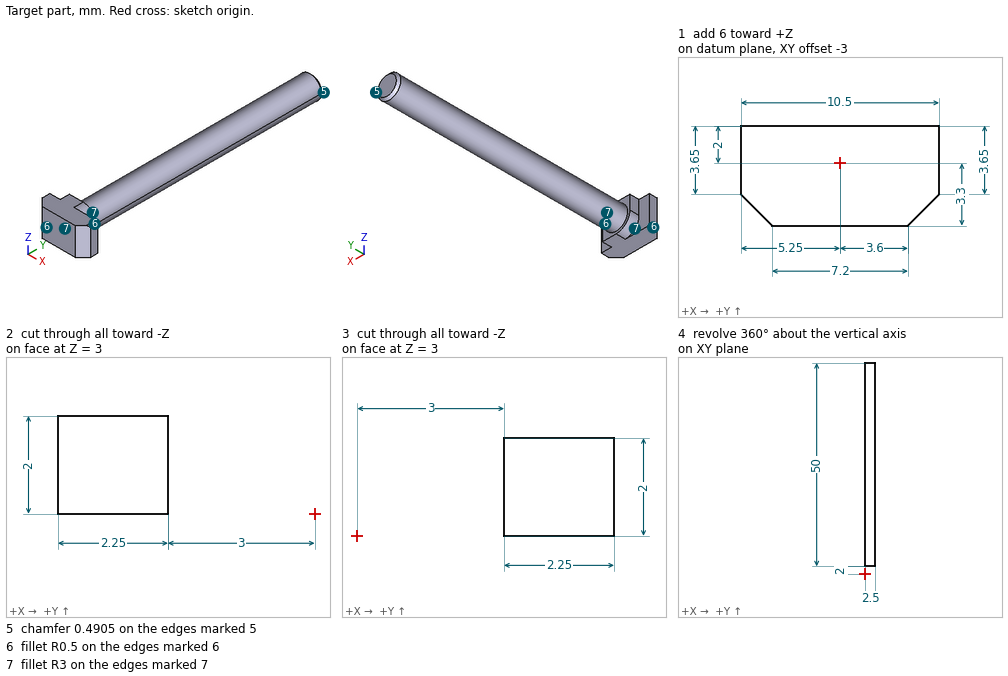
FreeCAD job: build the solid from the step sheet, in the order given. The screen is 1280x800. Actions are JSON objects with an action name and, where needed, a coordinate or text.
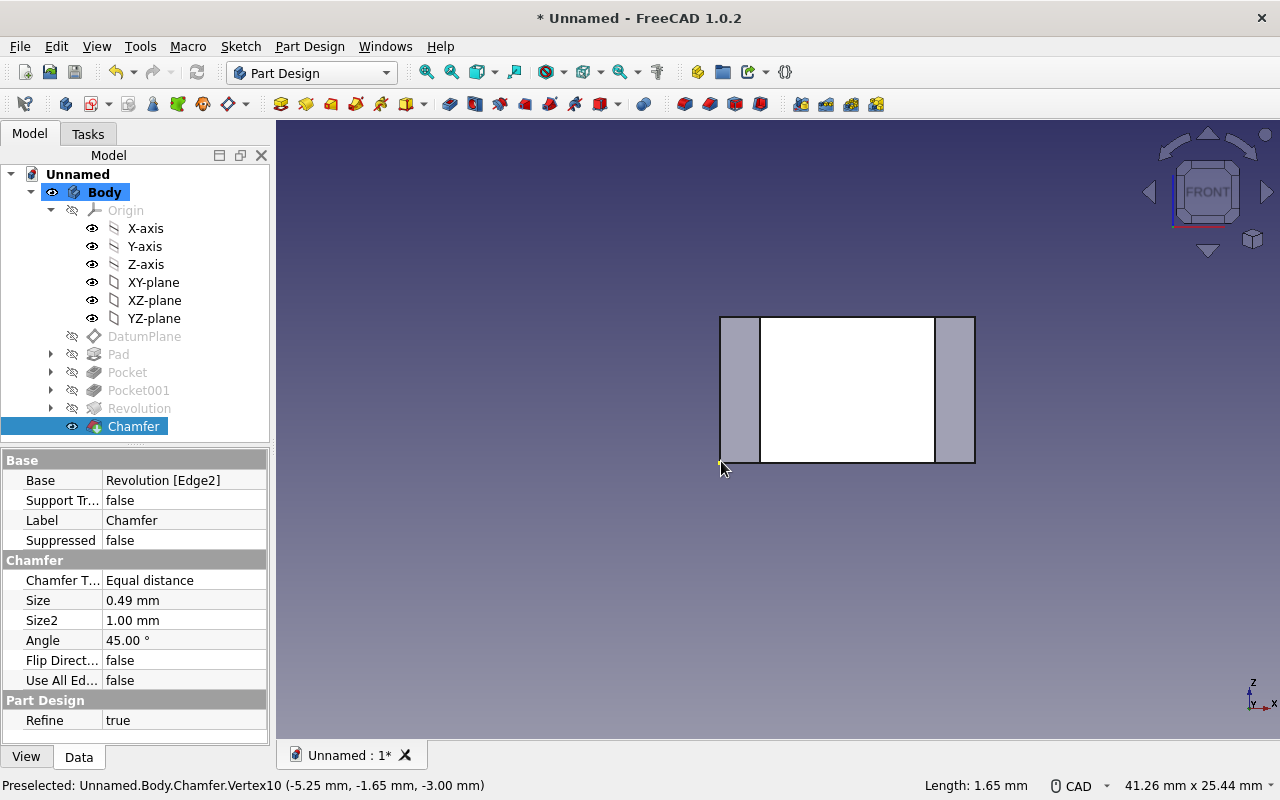
{"action": "key", "text": "v f"}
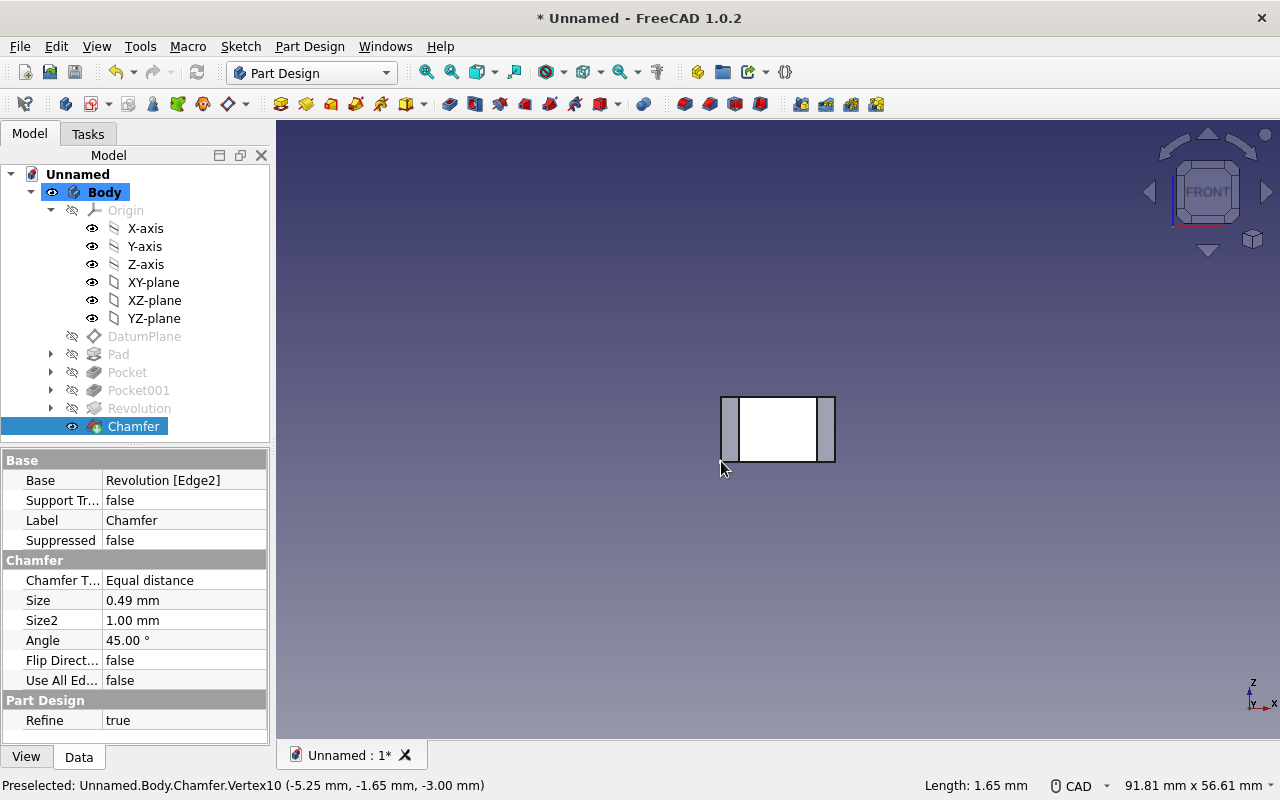
{"action": "key", "text": "3"}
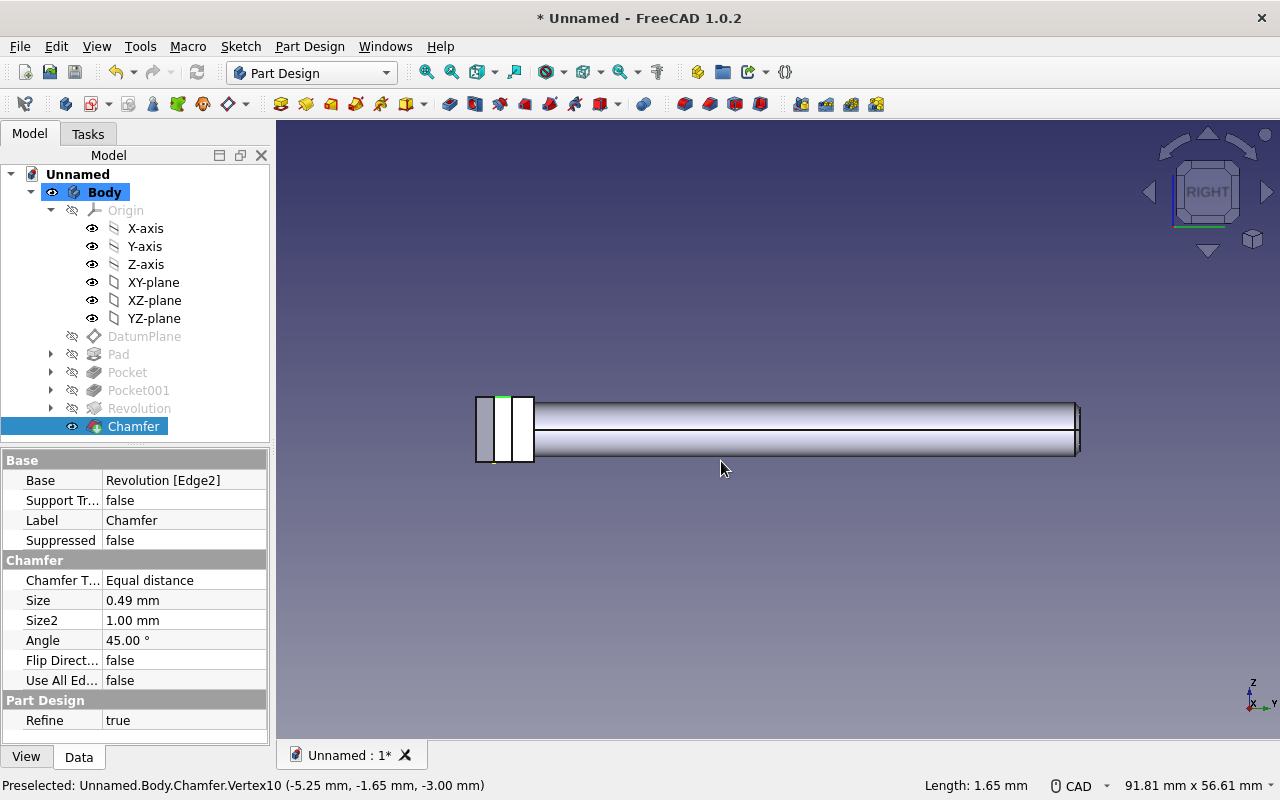
{"action": "scroll", "coordinate": [503, 461], "scroll_direction": "up", "scroll_amount": 4}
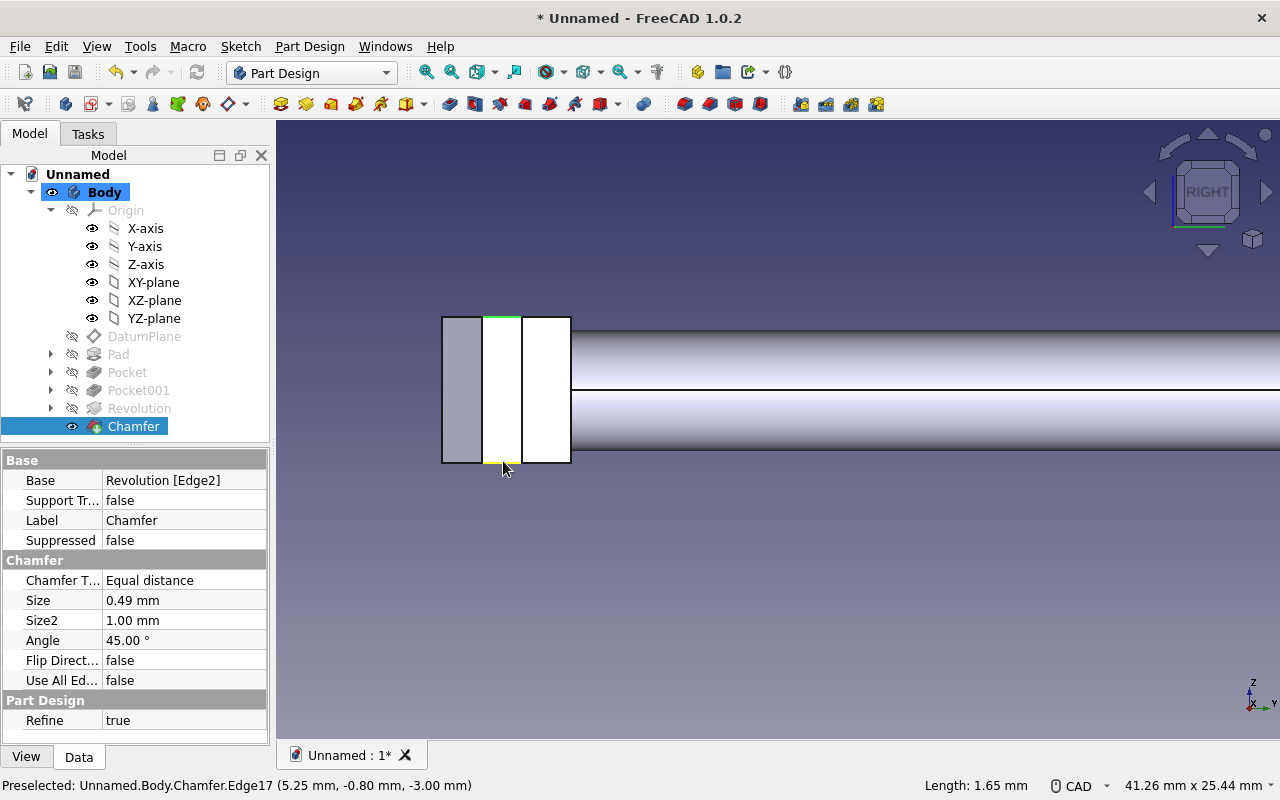
{"action": "key", "text": "v f"}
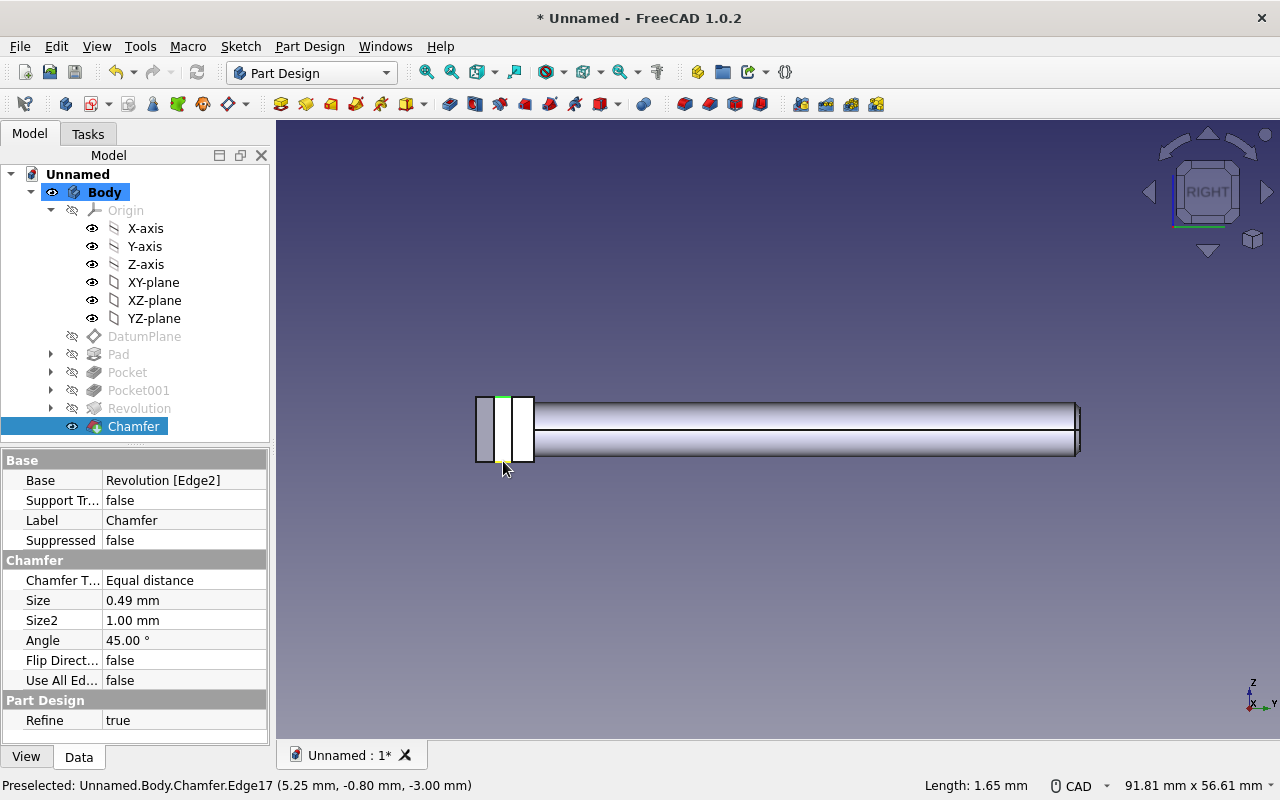
{"action": "key", "text": "5"}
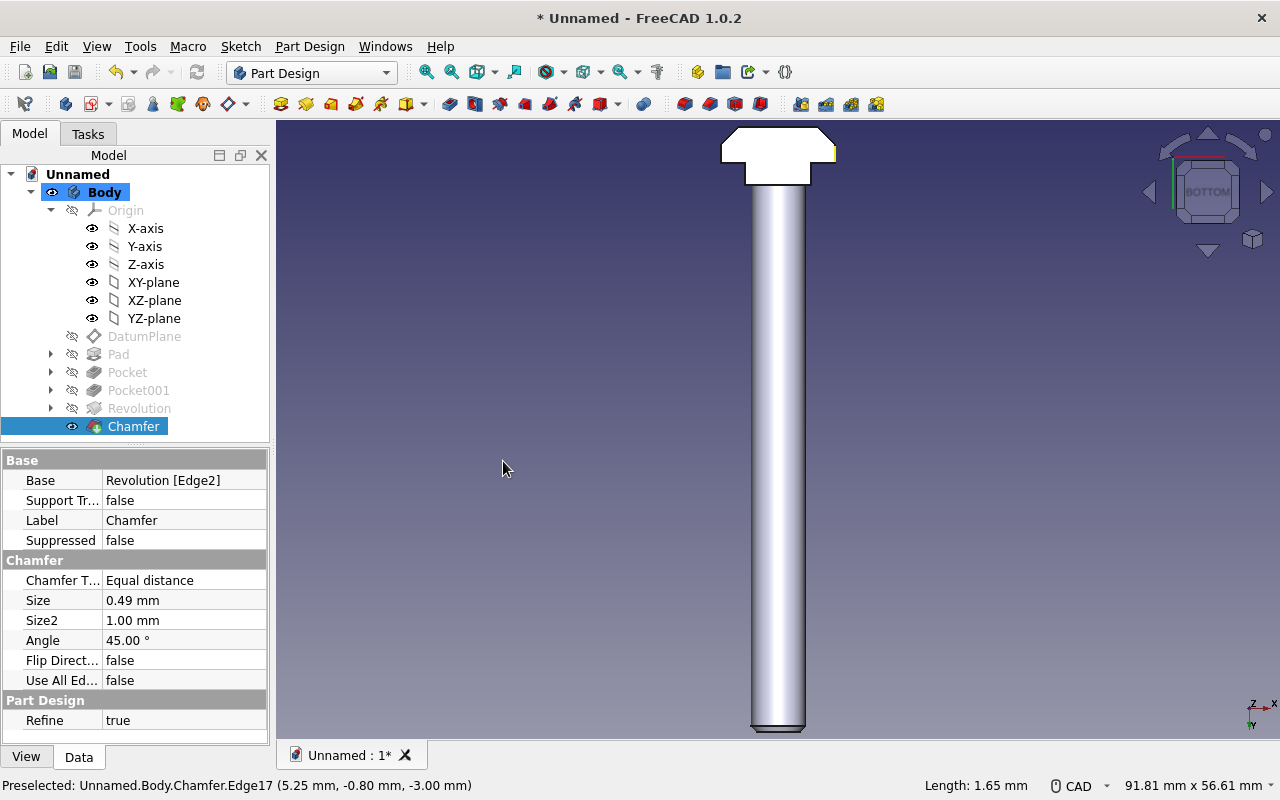
{"action": "left_click", "coordinate": [721, 153], "text": "ctrl"}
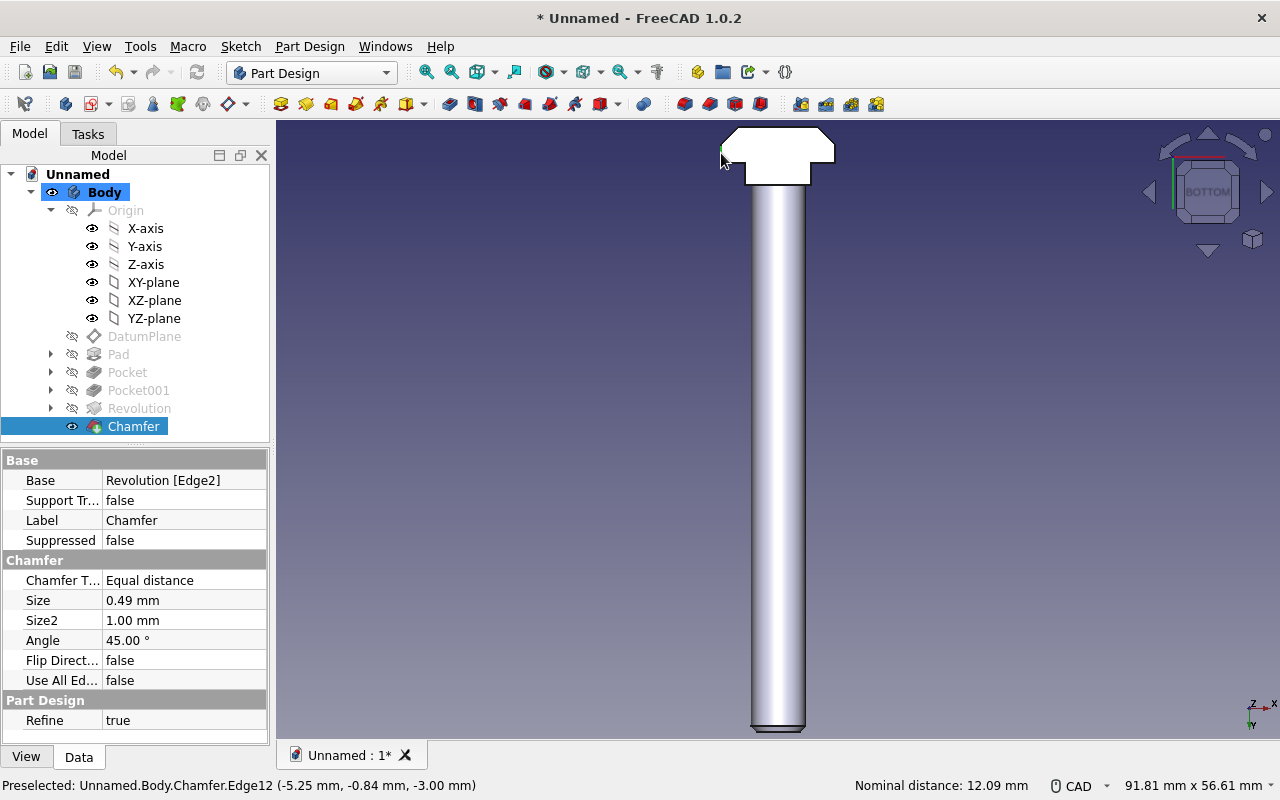
{"action": "left_click", "coordinate": [685, 104]}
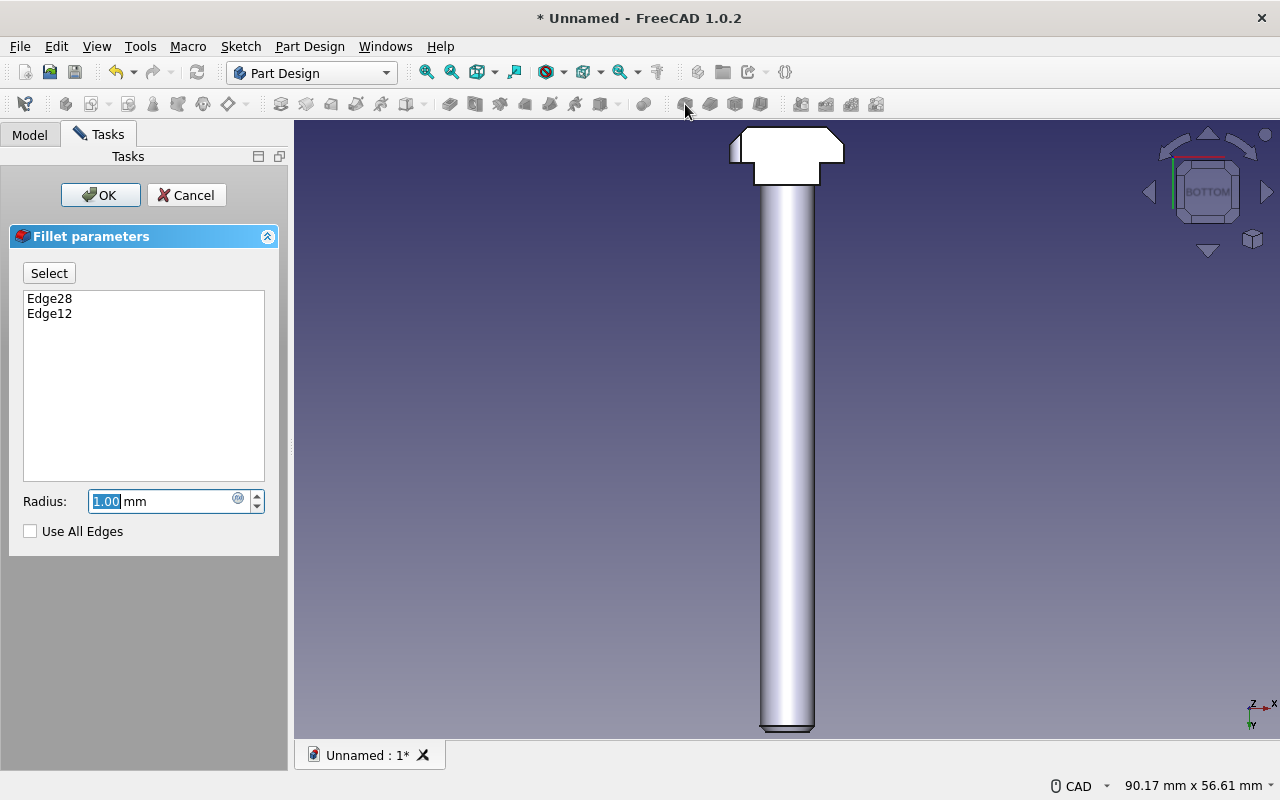
{"action": "type", "text": "0.5"}
{"action": "key", "text": "Tab"}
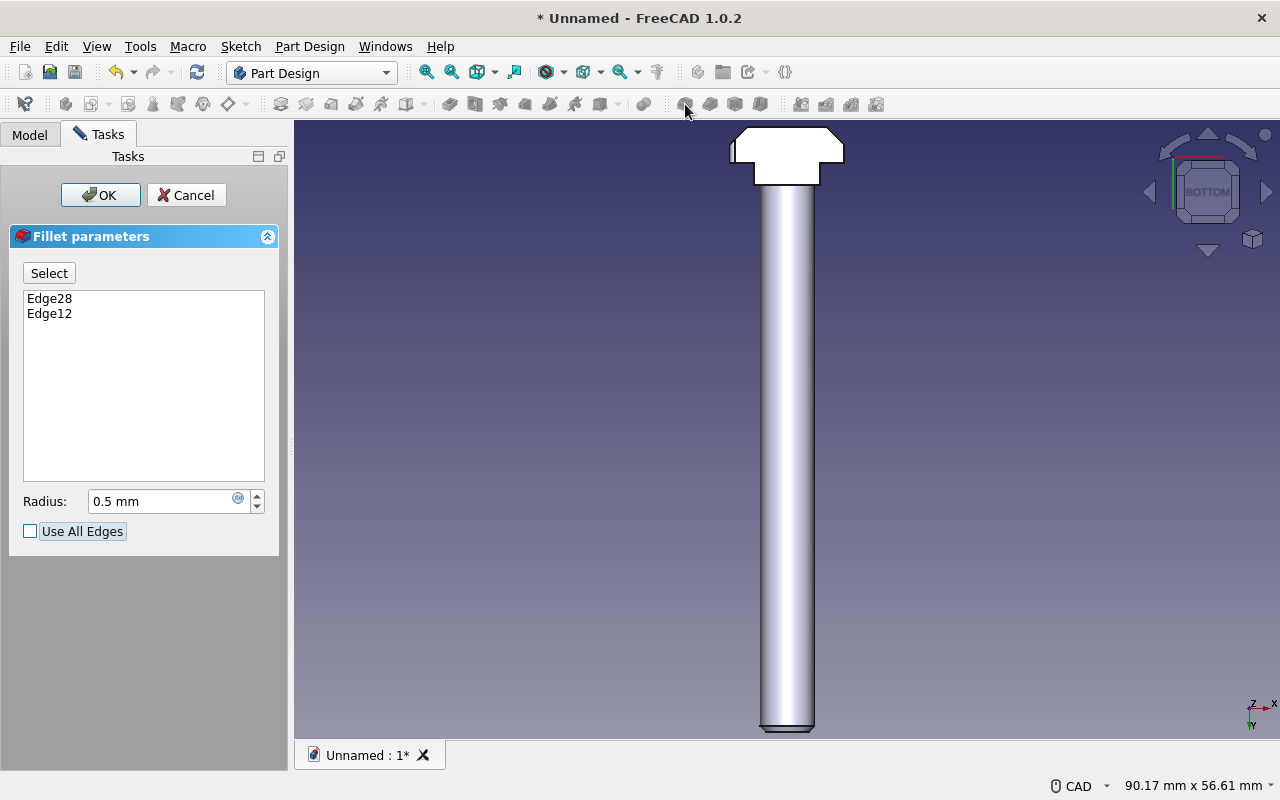
{"action": "left_click", "coordinate": [101, 195]}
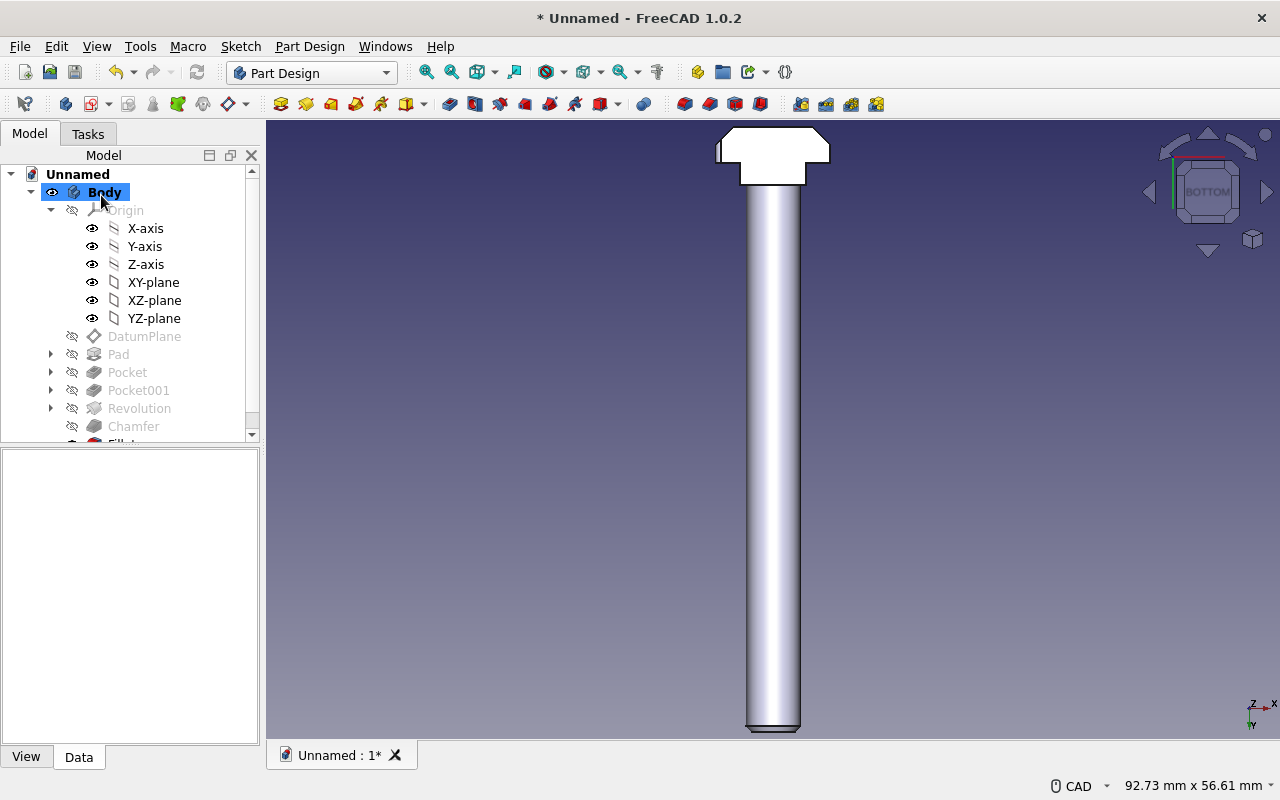
{"action": "left_click", "coordinate": [740, 173]}